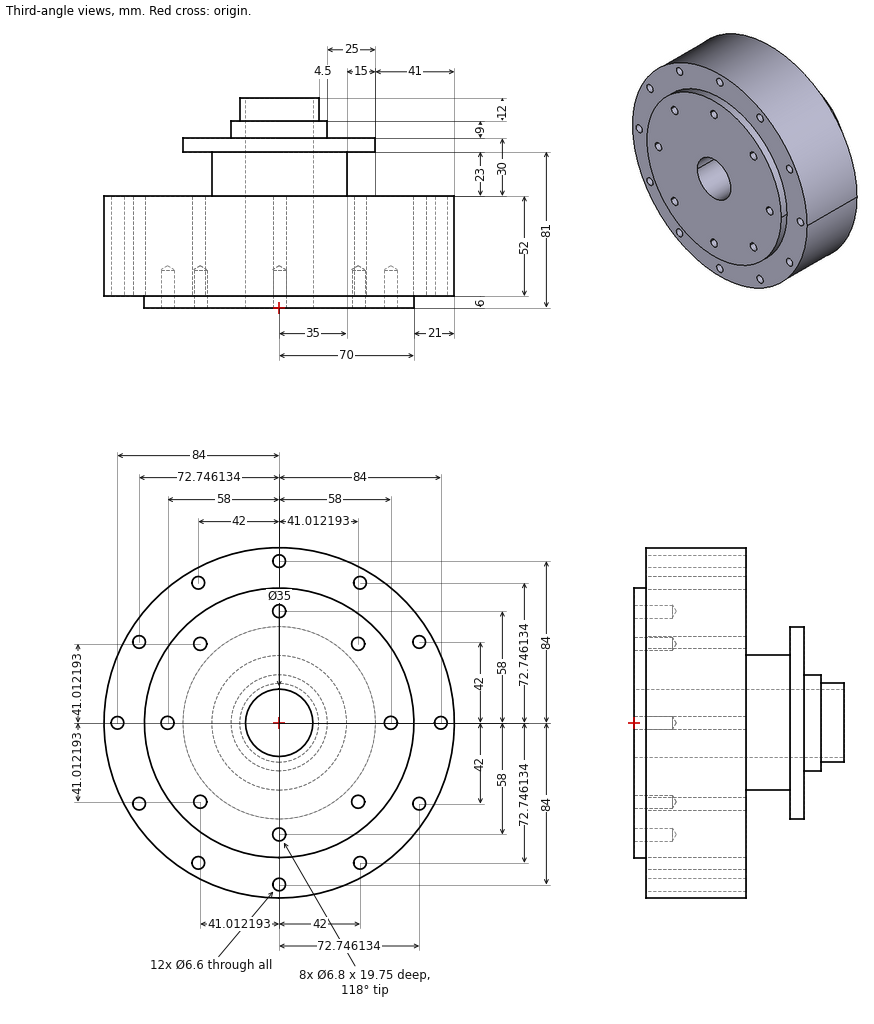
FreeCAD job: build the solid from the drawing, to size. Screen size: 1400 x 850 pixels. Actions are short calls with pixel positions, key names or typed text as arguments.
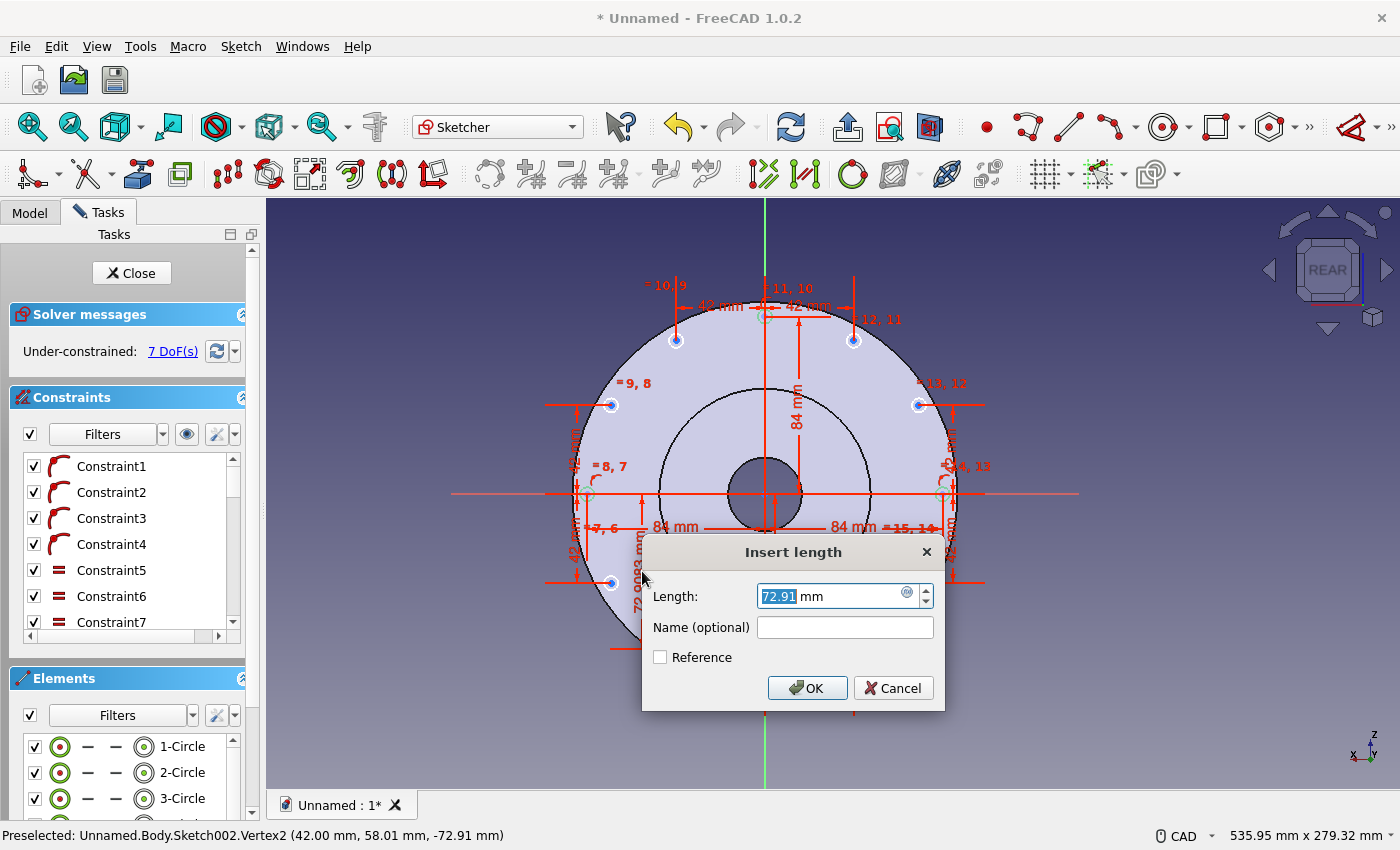
text(72.746134)
key(Return)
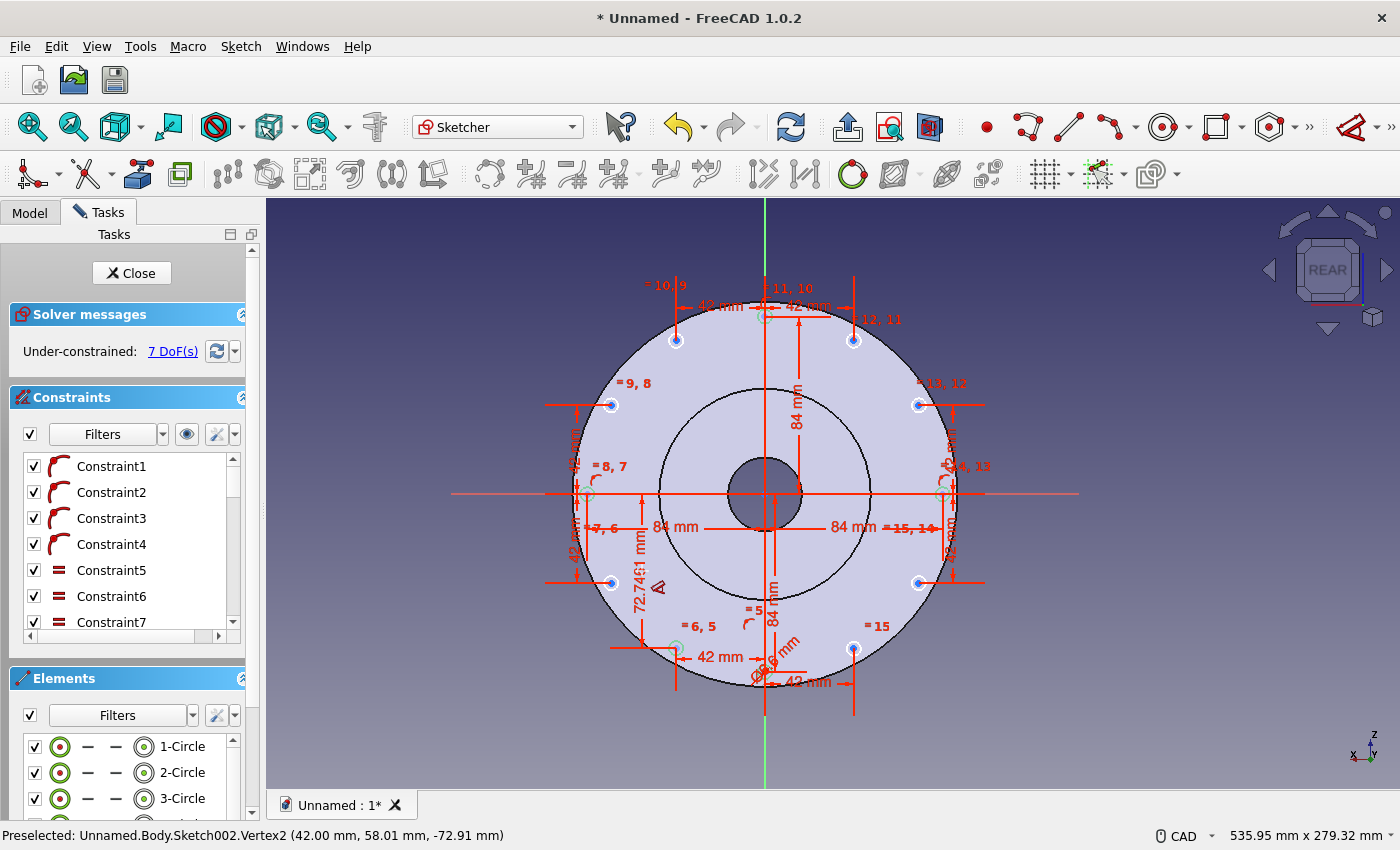
click(611, 583)
click(688, 617)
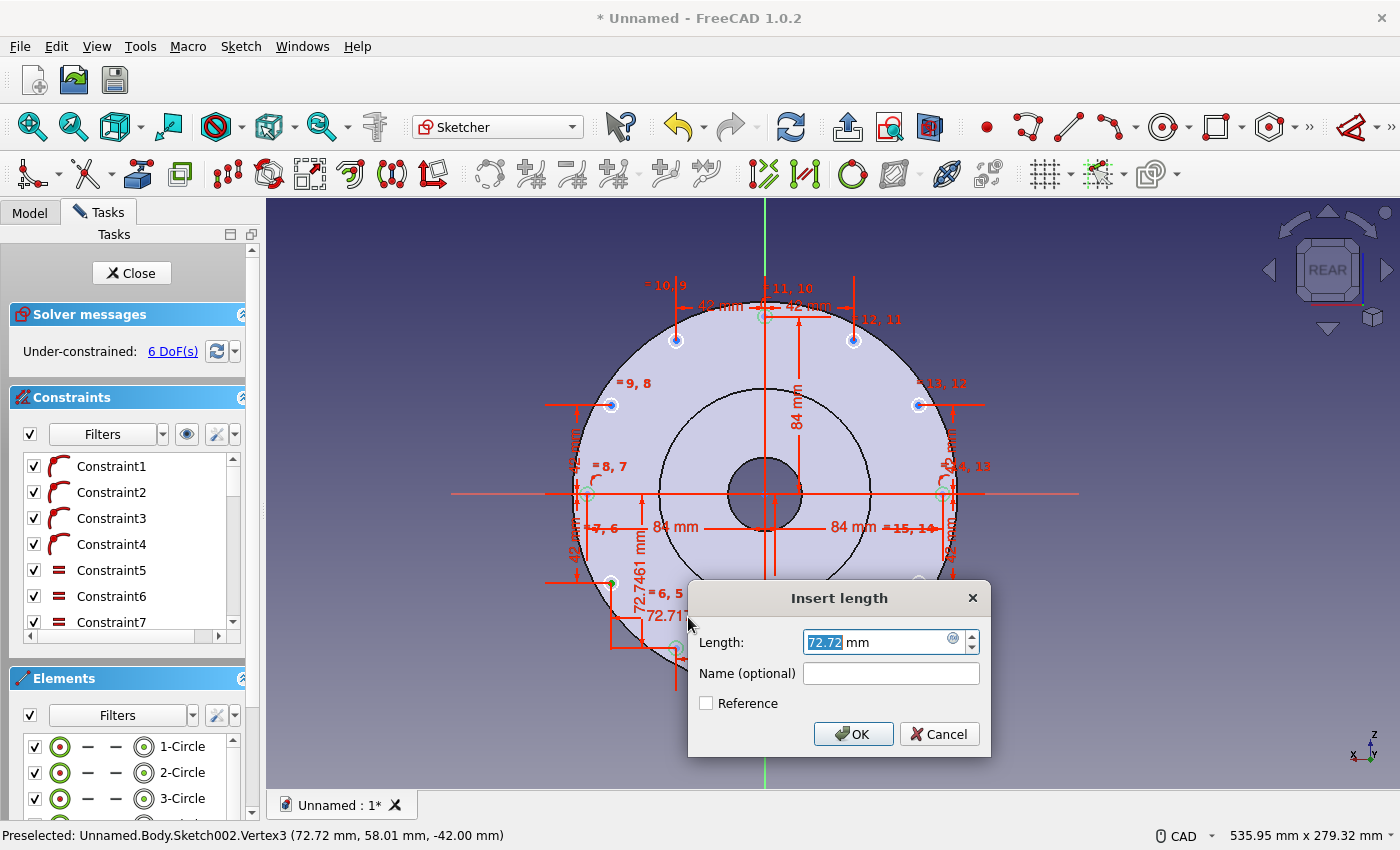
text(72.746134)
key(Return)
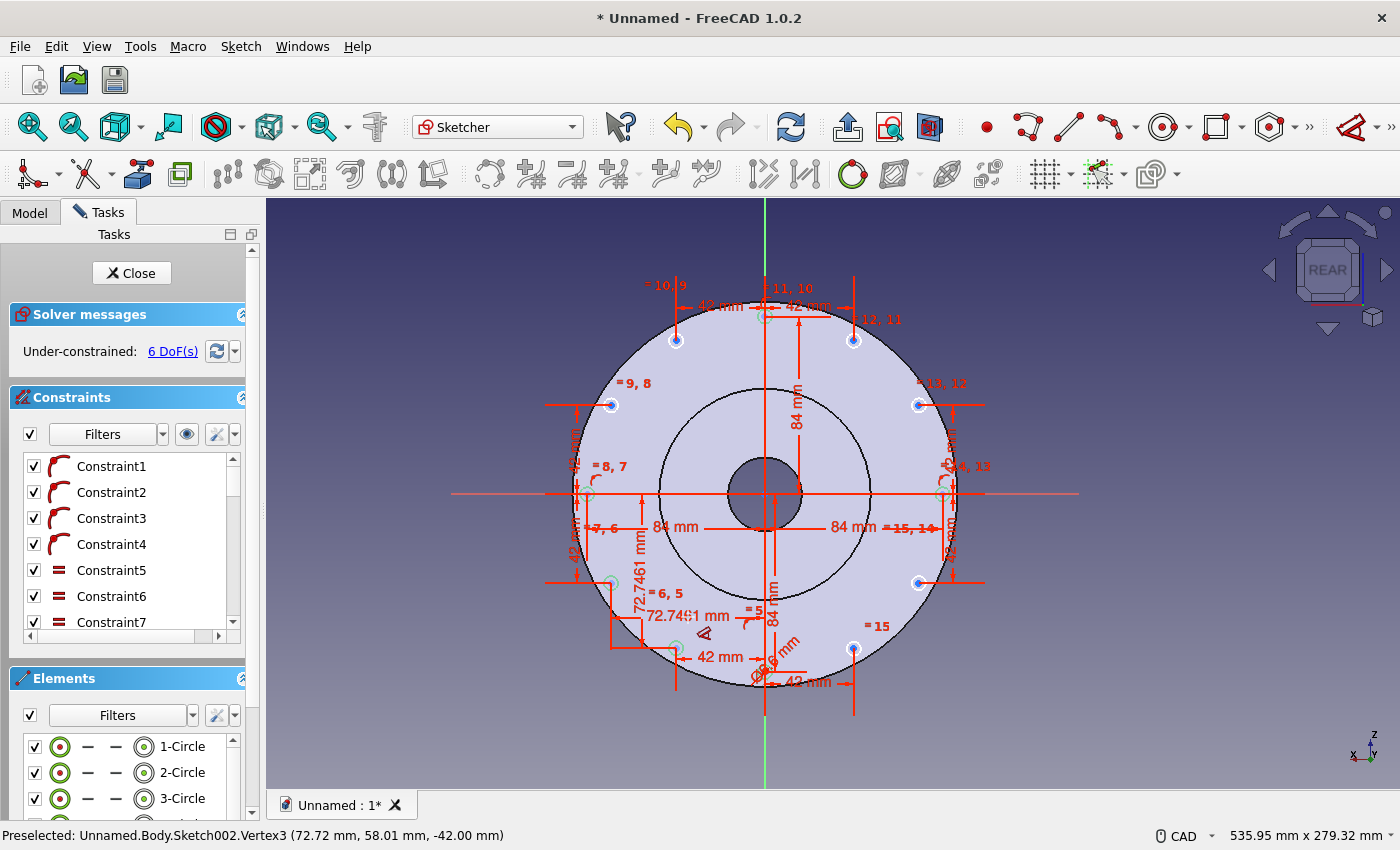
click(611, 405)
click(688, 371)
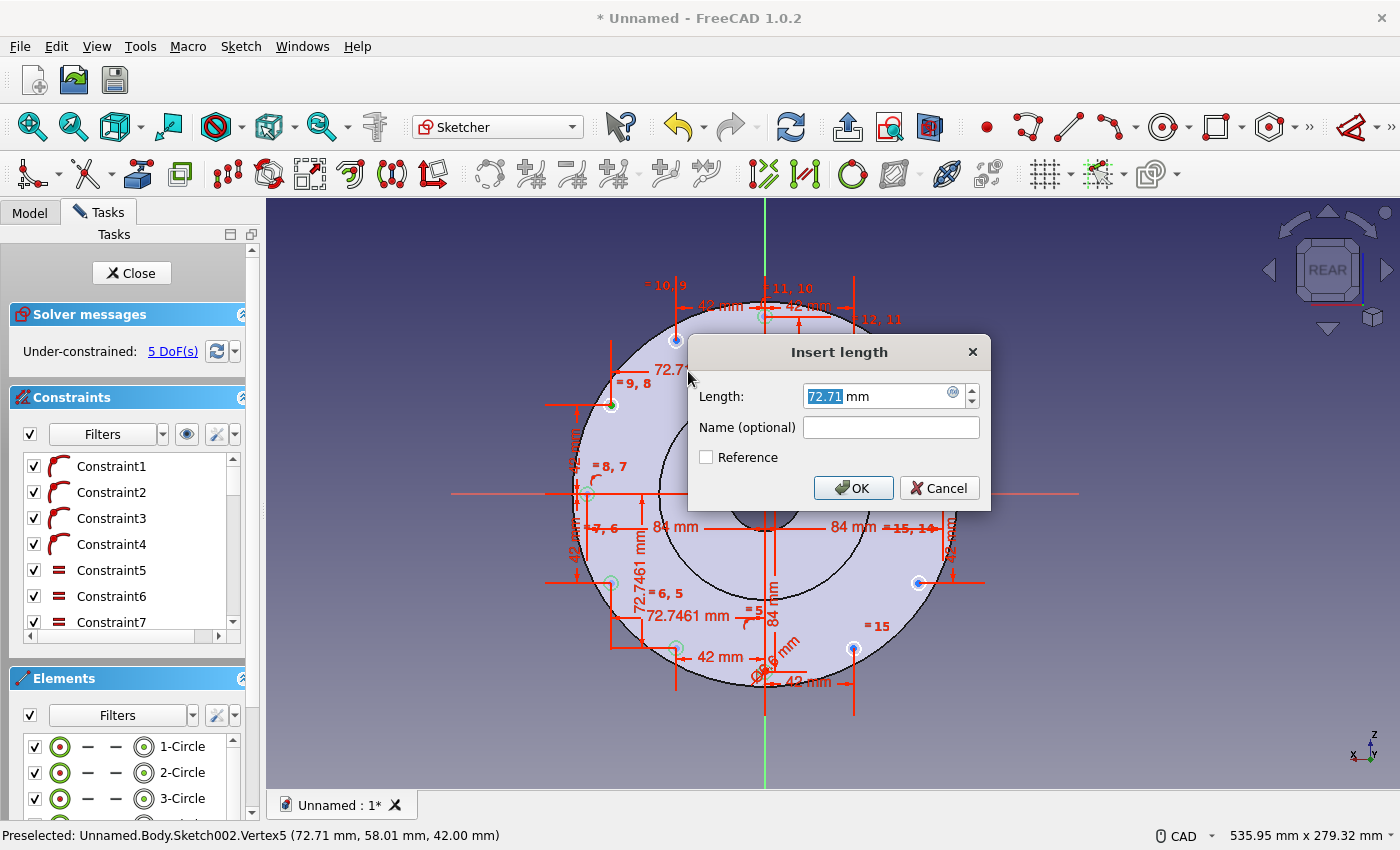
text(72.746134)
key(Return)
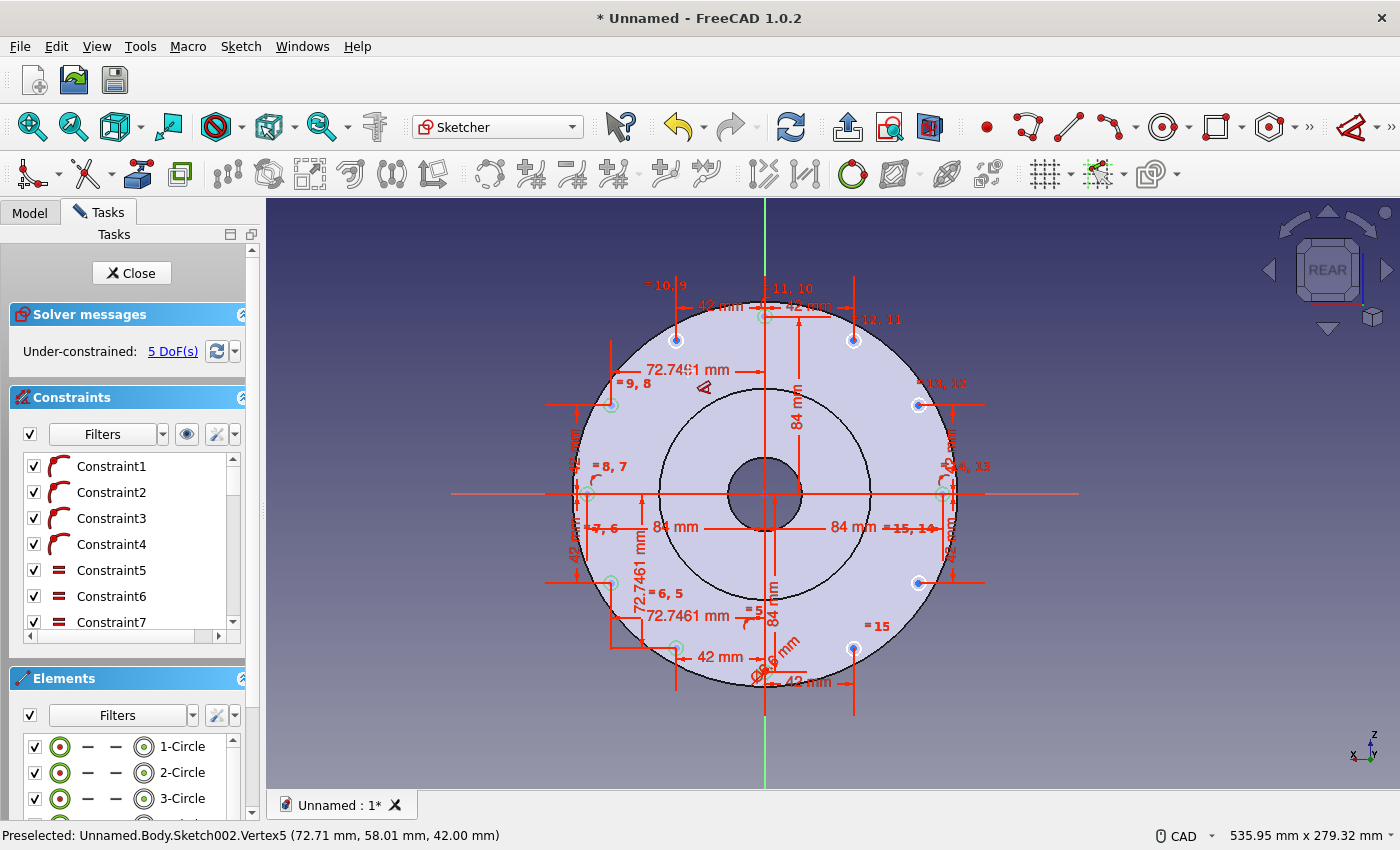
click(676, 341)
click(642, 417)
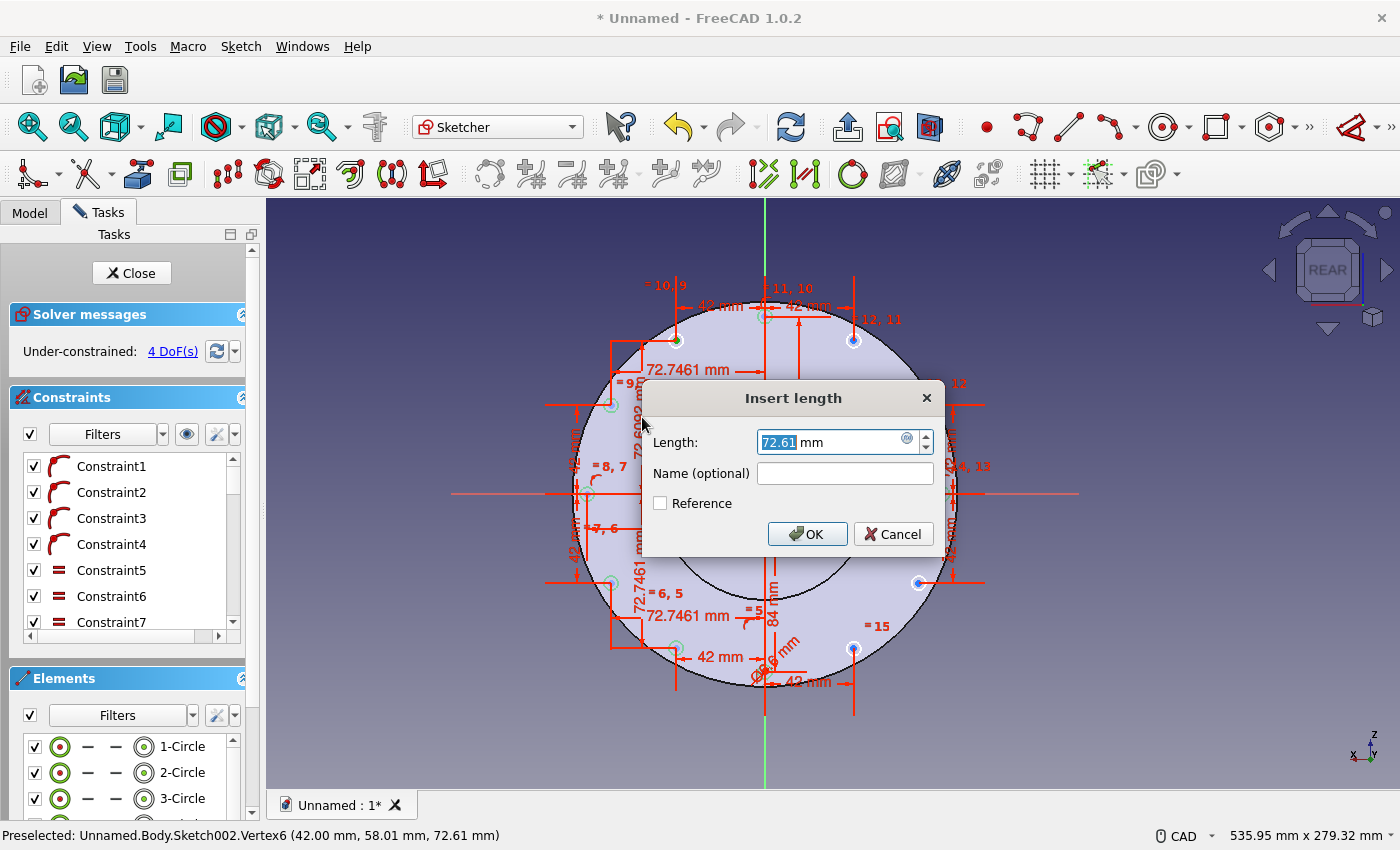
text(72.746134)
key(Return)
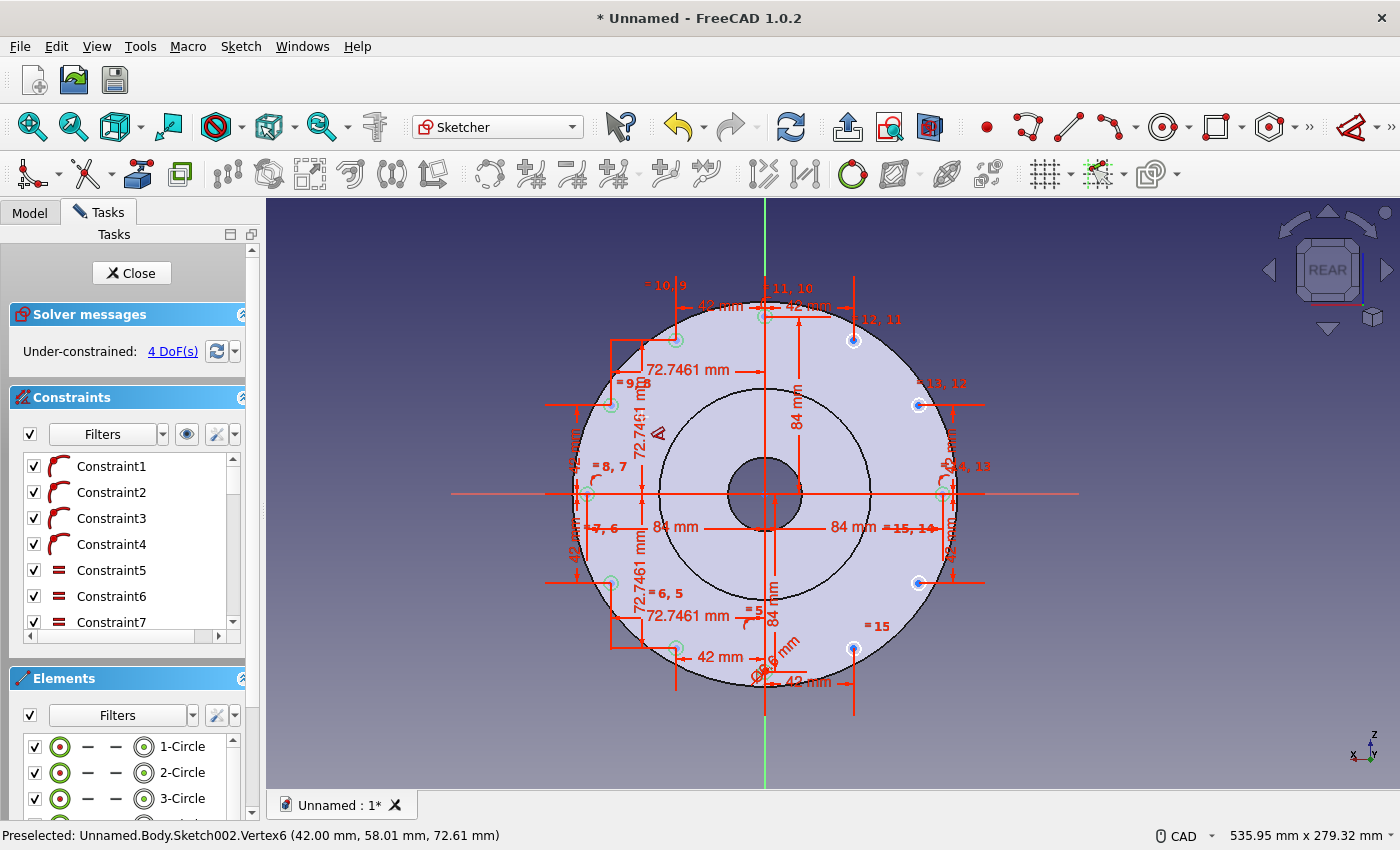
click(854, 341)
click(888, 417)